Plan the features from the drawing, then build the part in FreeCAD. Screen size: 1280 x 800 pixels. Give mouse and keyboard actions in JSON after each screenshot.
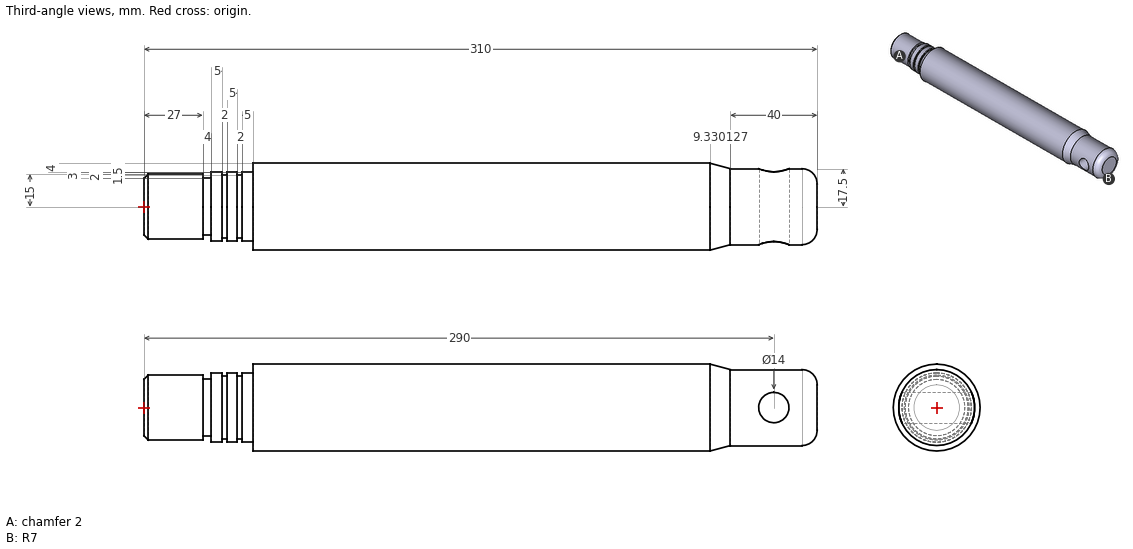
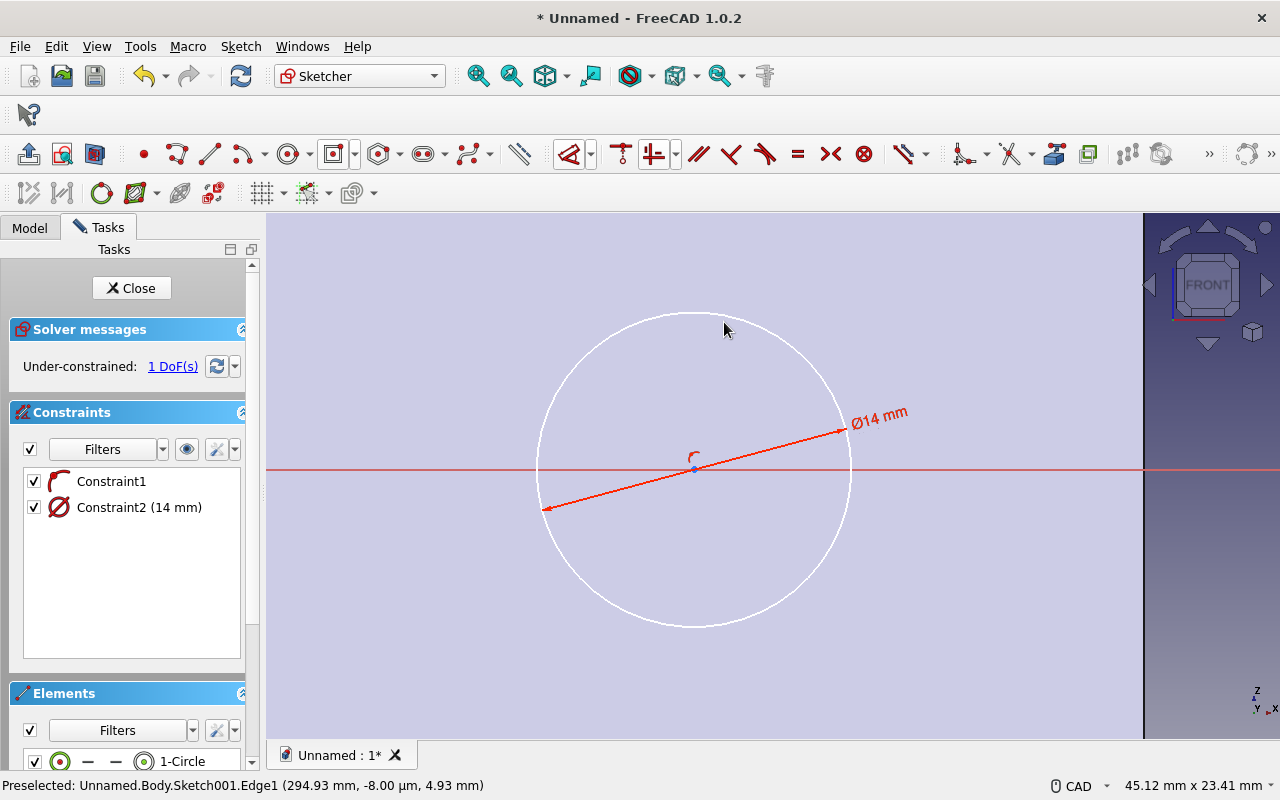
{"action": "left_click", "coordinate": [694, 470]}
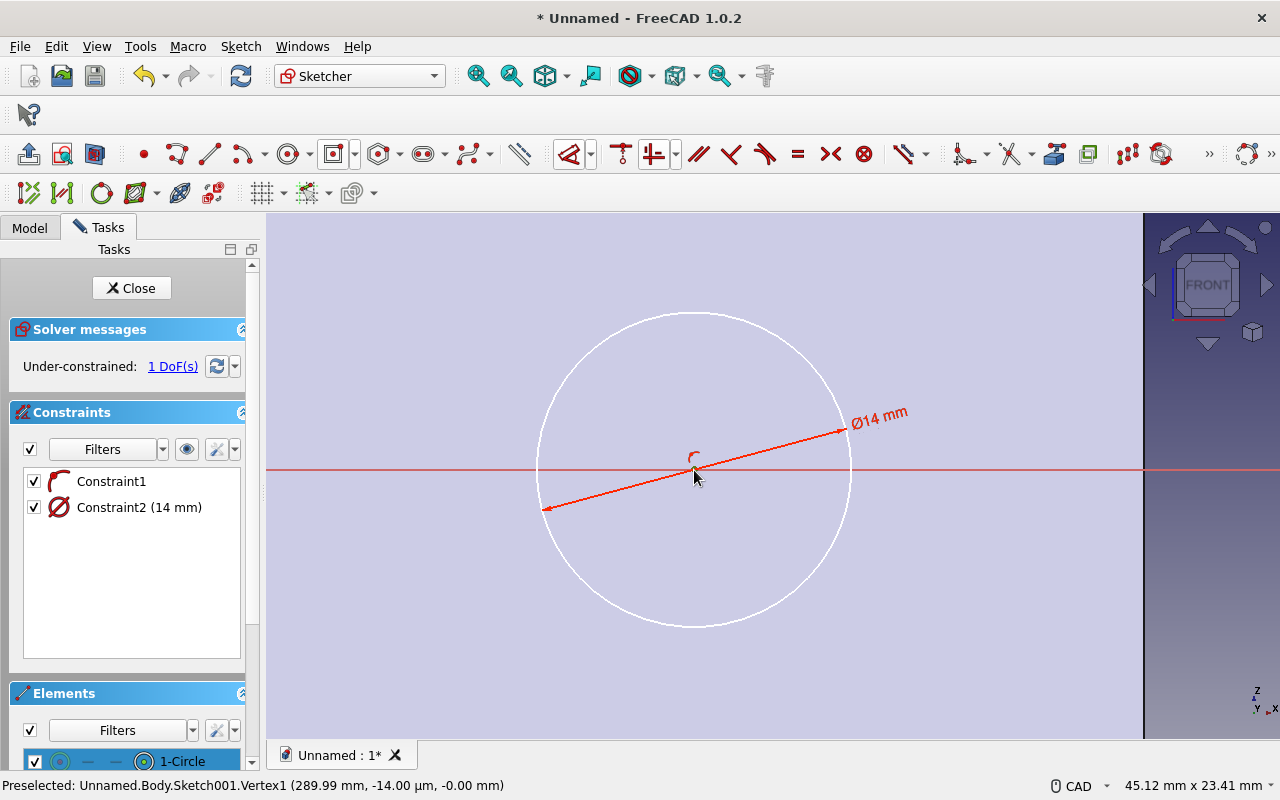
{"action": "left_click", "coordinate": [590, 154]}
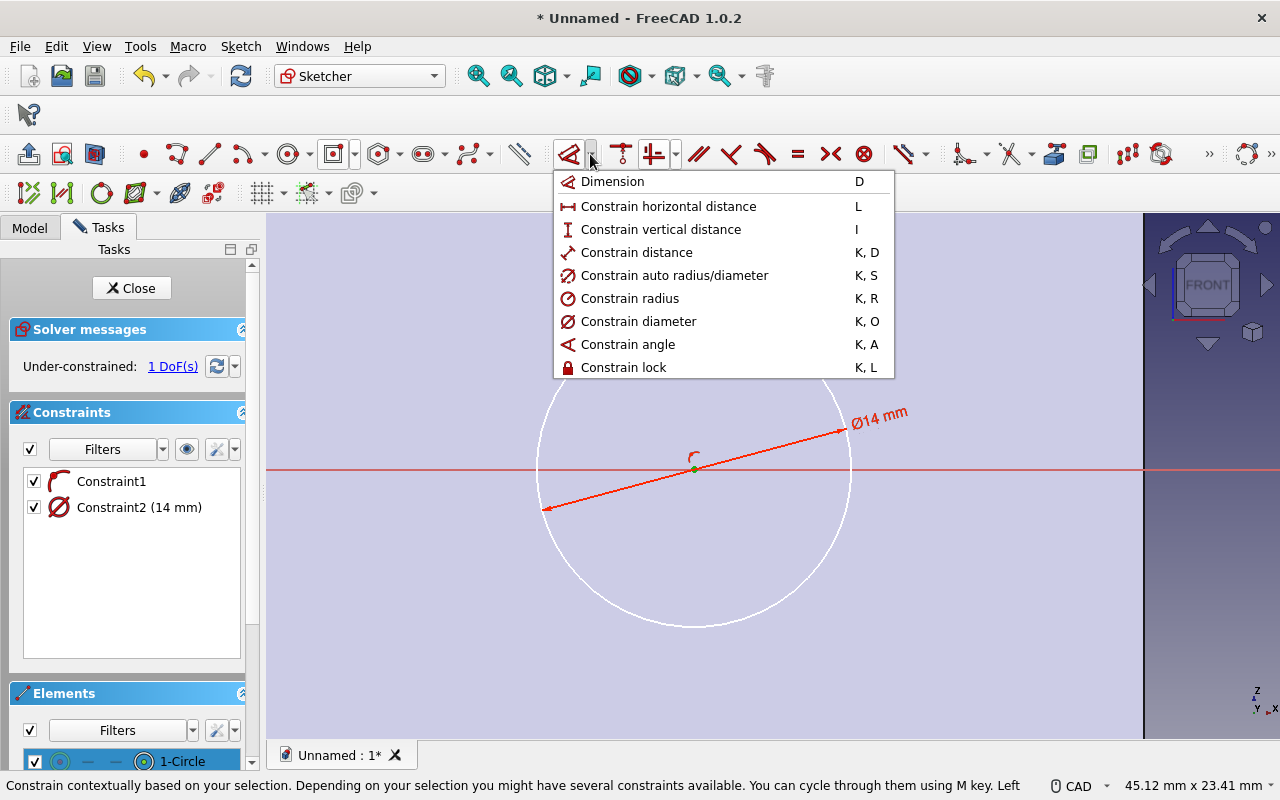
{"action": "left_click", "coordinate": [724, 206]}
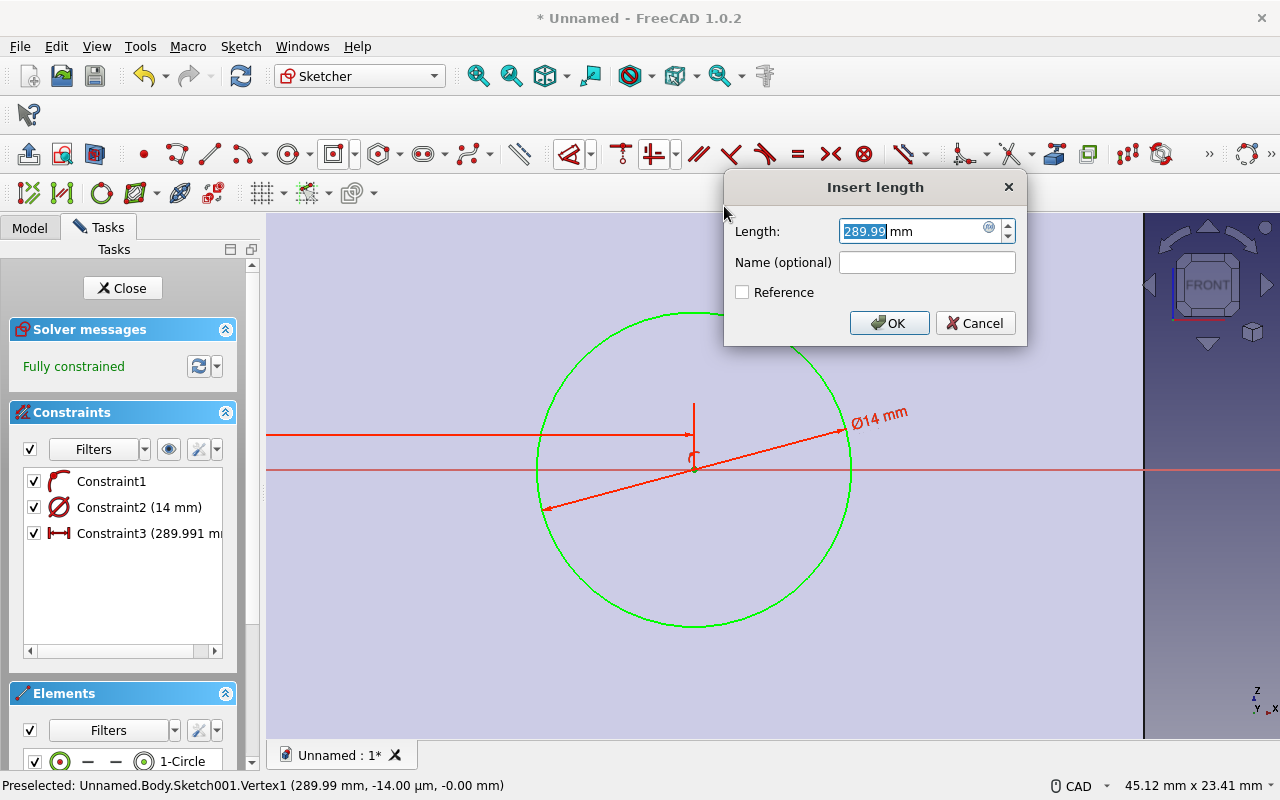
{"action": "type", "text": "290"}
{"action": "key", "text": "Return"}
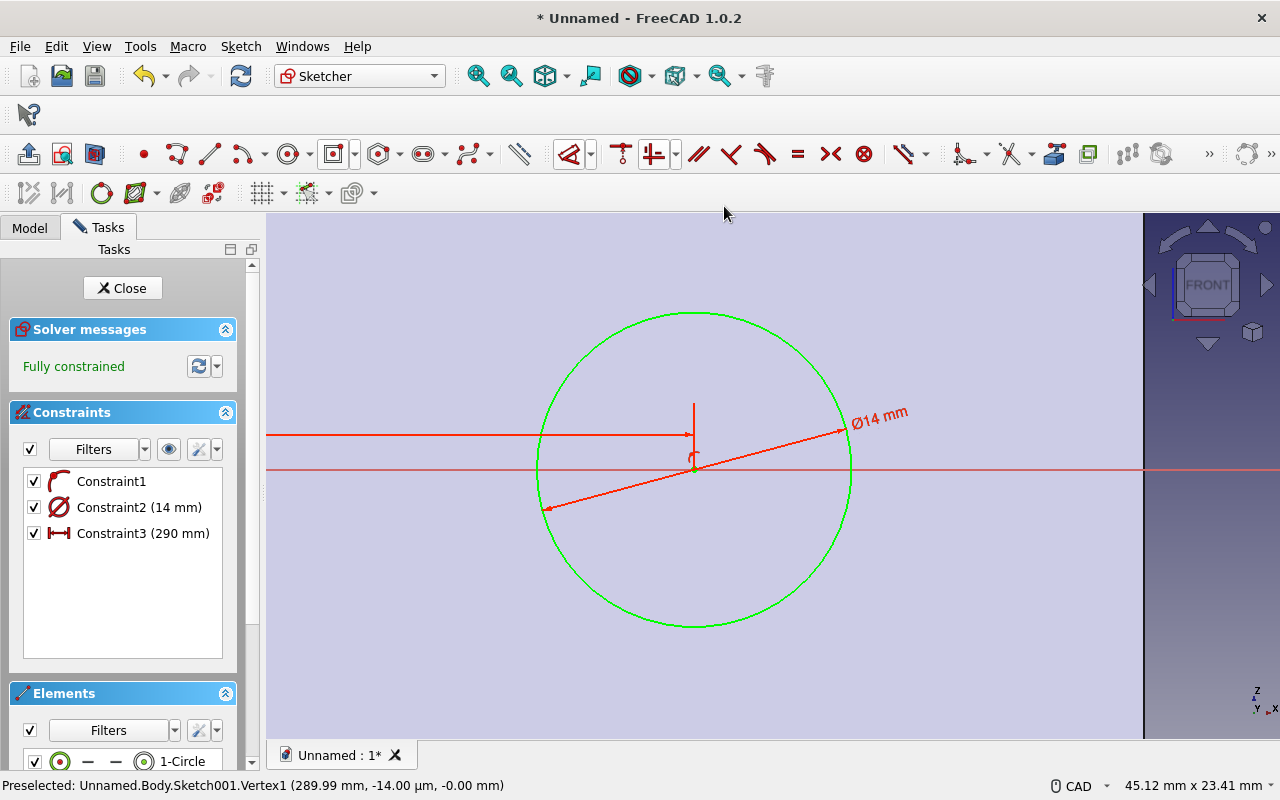
{"action": "left_click", "coordinate": [123, 288]}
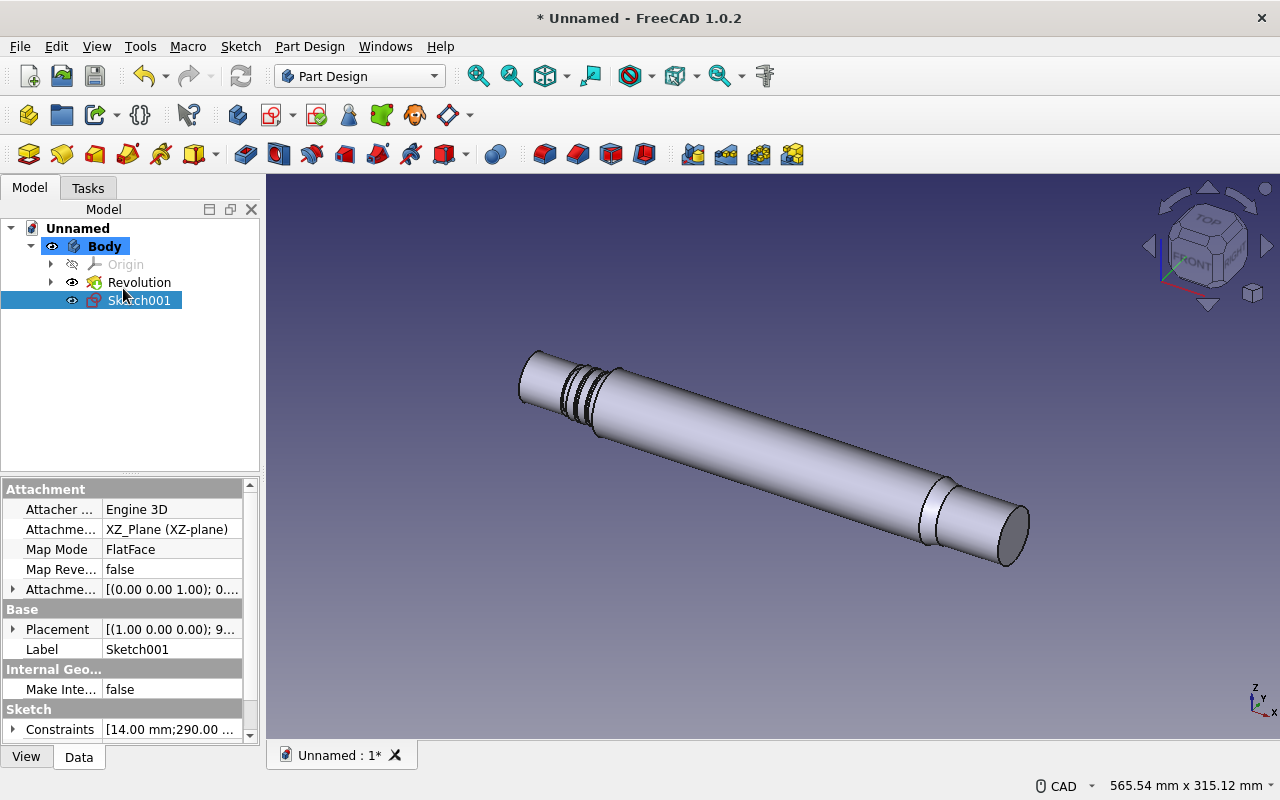
{"action": "left_click", "coordinate": [246, 154]}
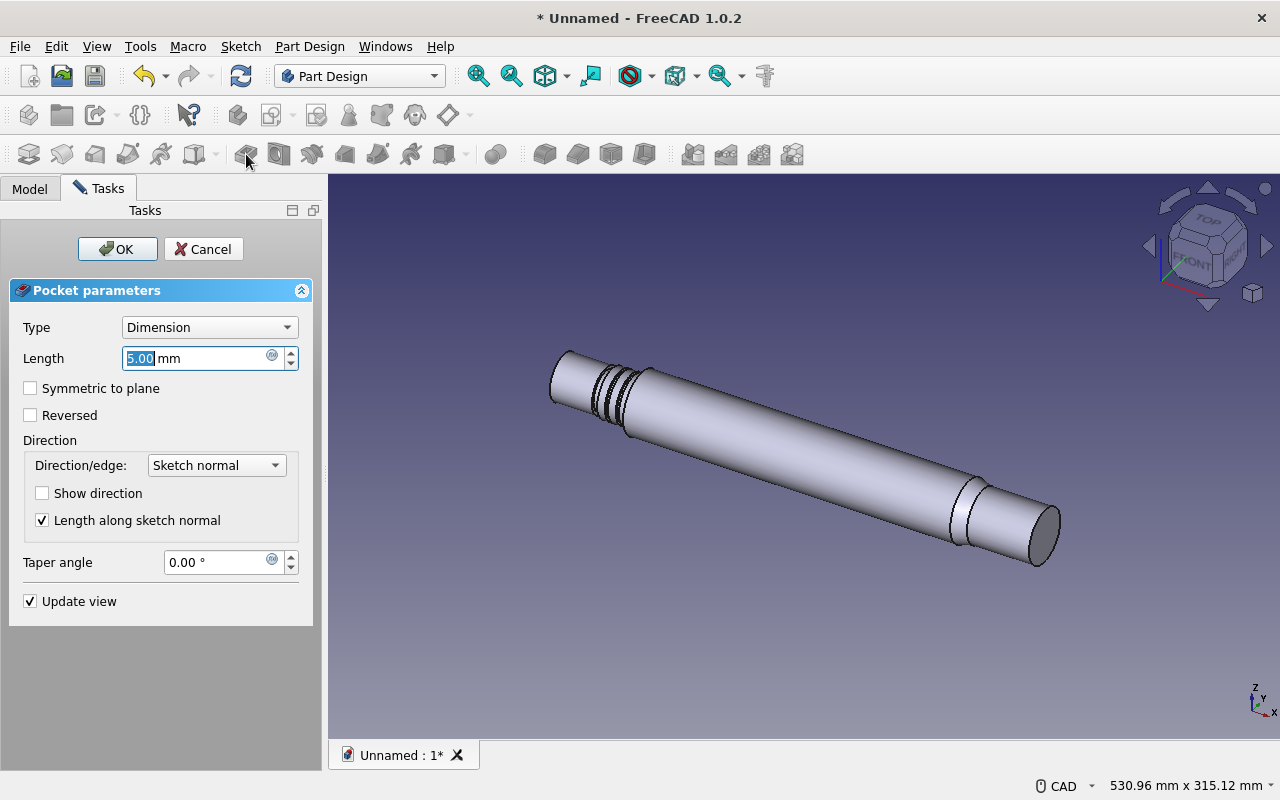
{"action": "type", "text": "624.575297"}
{"action": "key", "text": "Tab"}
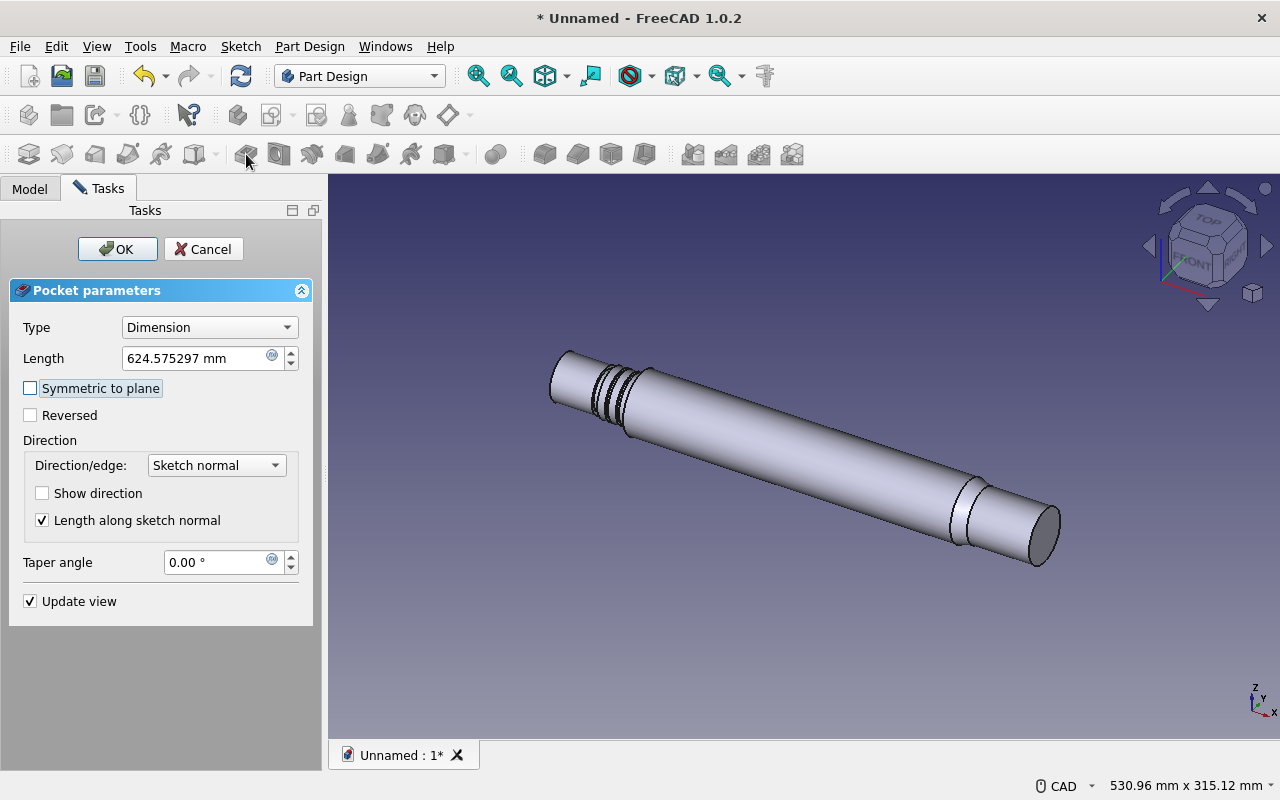
{"action": "left_click", "coordinate": [31, 388]}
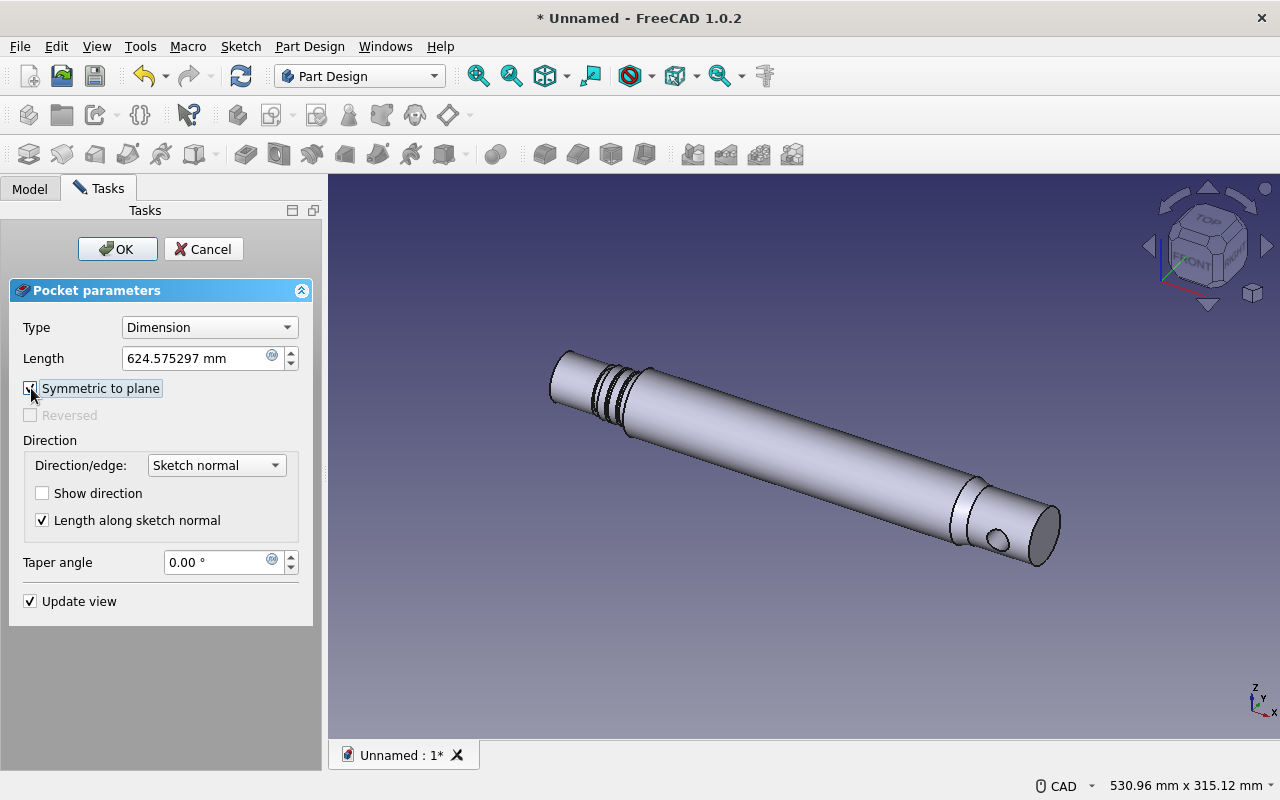
{"action": "left_click", "coordinate": [118, 249]}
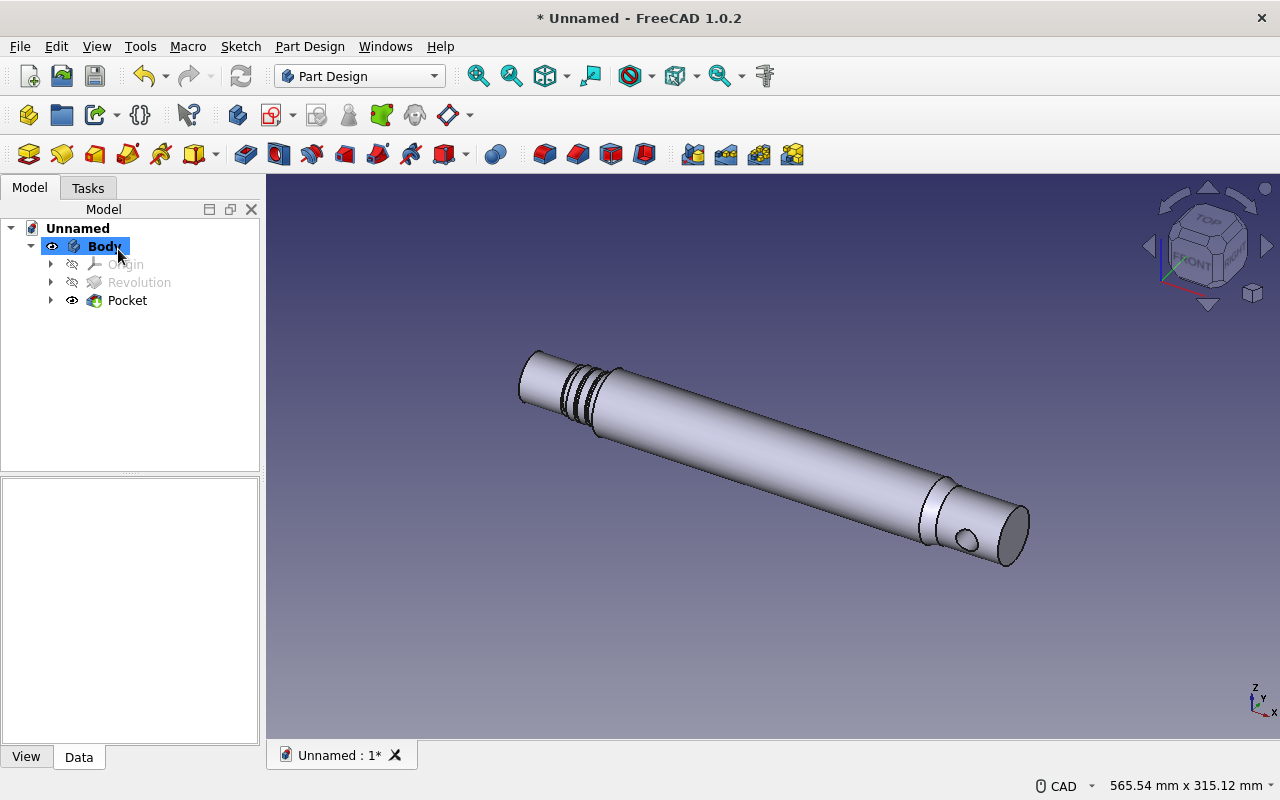
{"action": "left_click", "coordinate": [521, 400]}